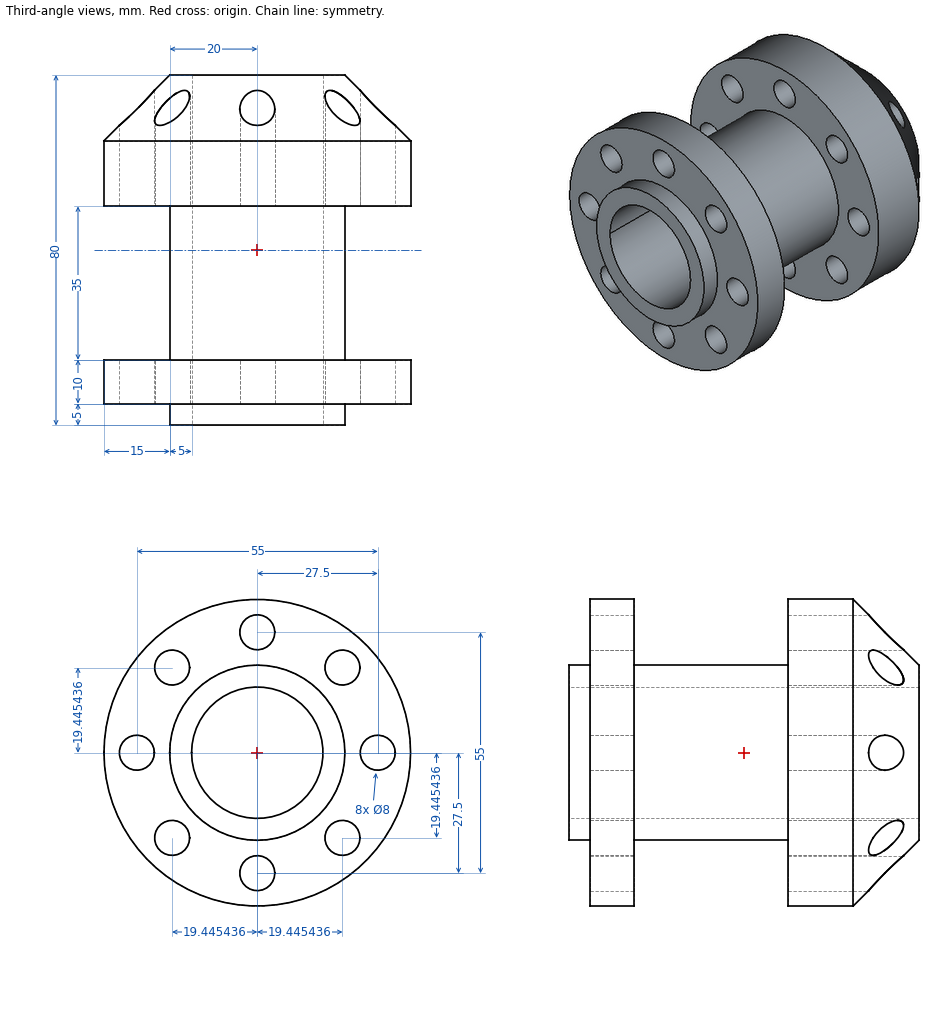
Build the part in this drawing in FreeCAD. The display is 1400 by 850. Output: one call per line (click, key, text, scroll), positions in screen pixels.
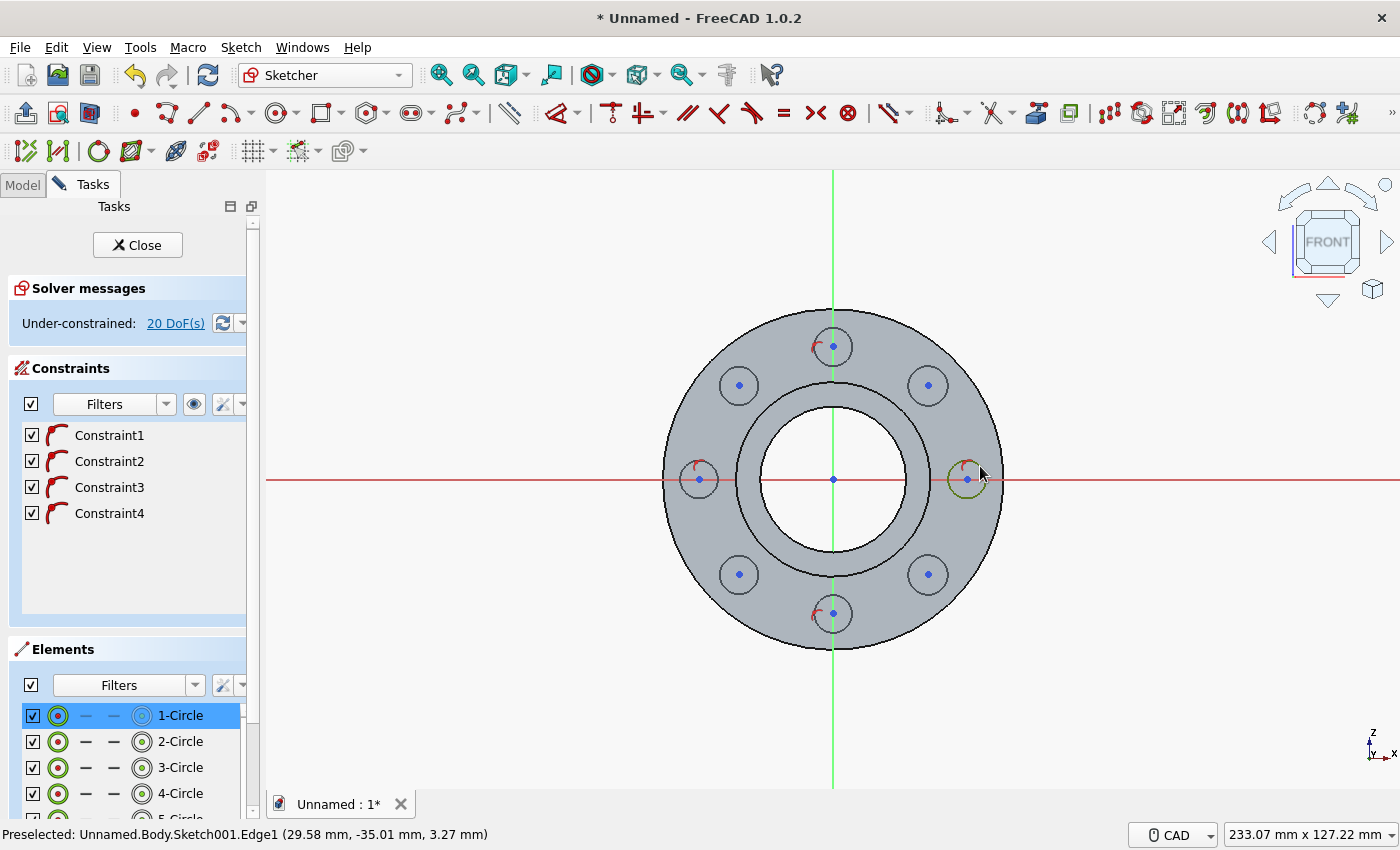
click(942, 561)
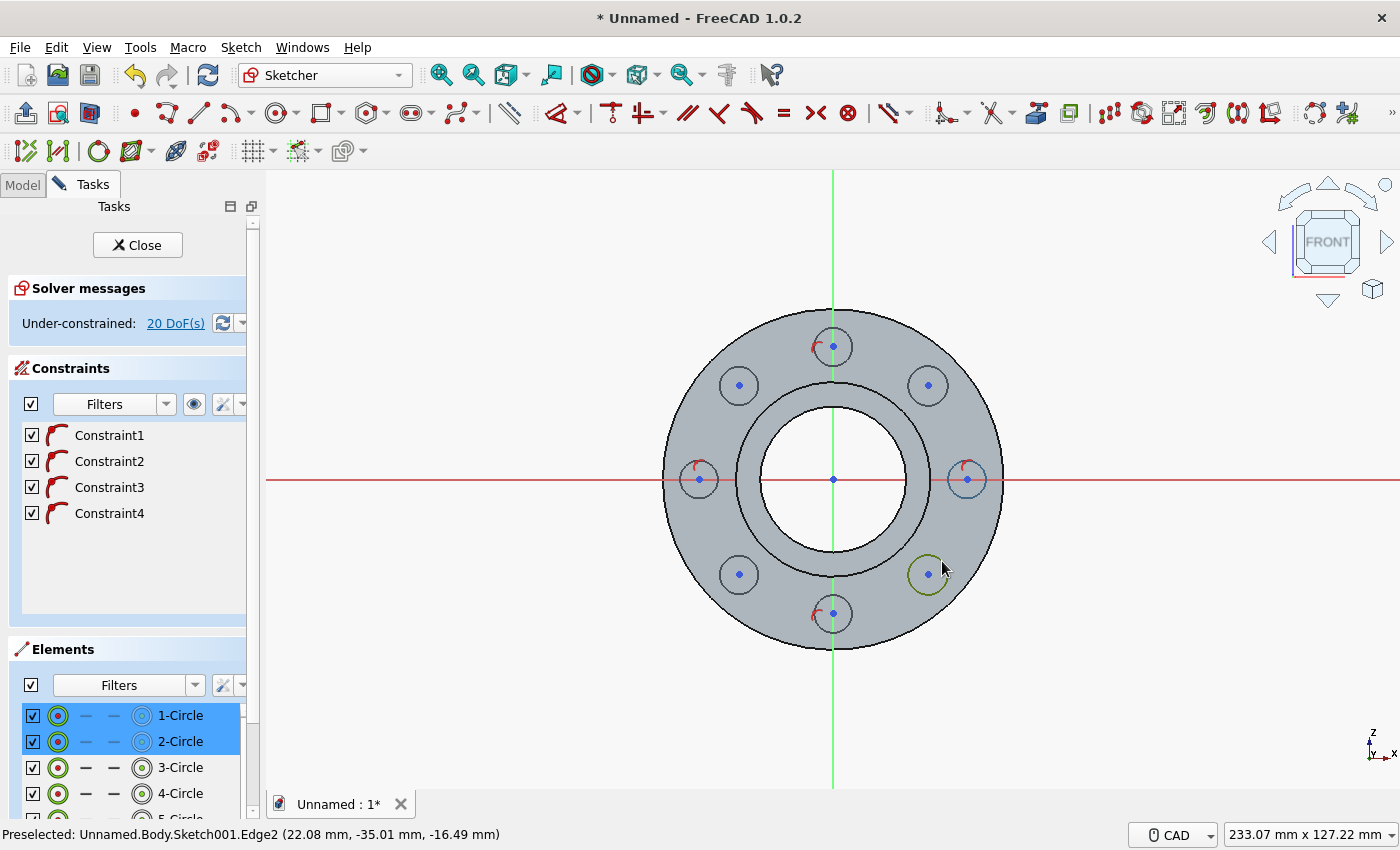
click(846, 601)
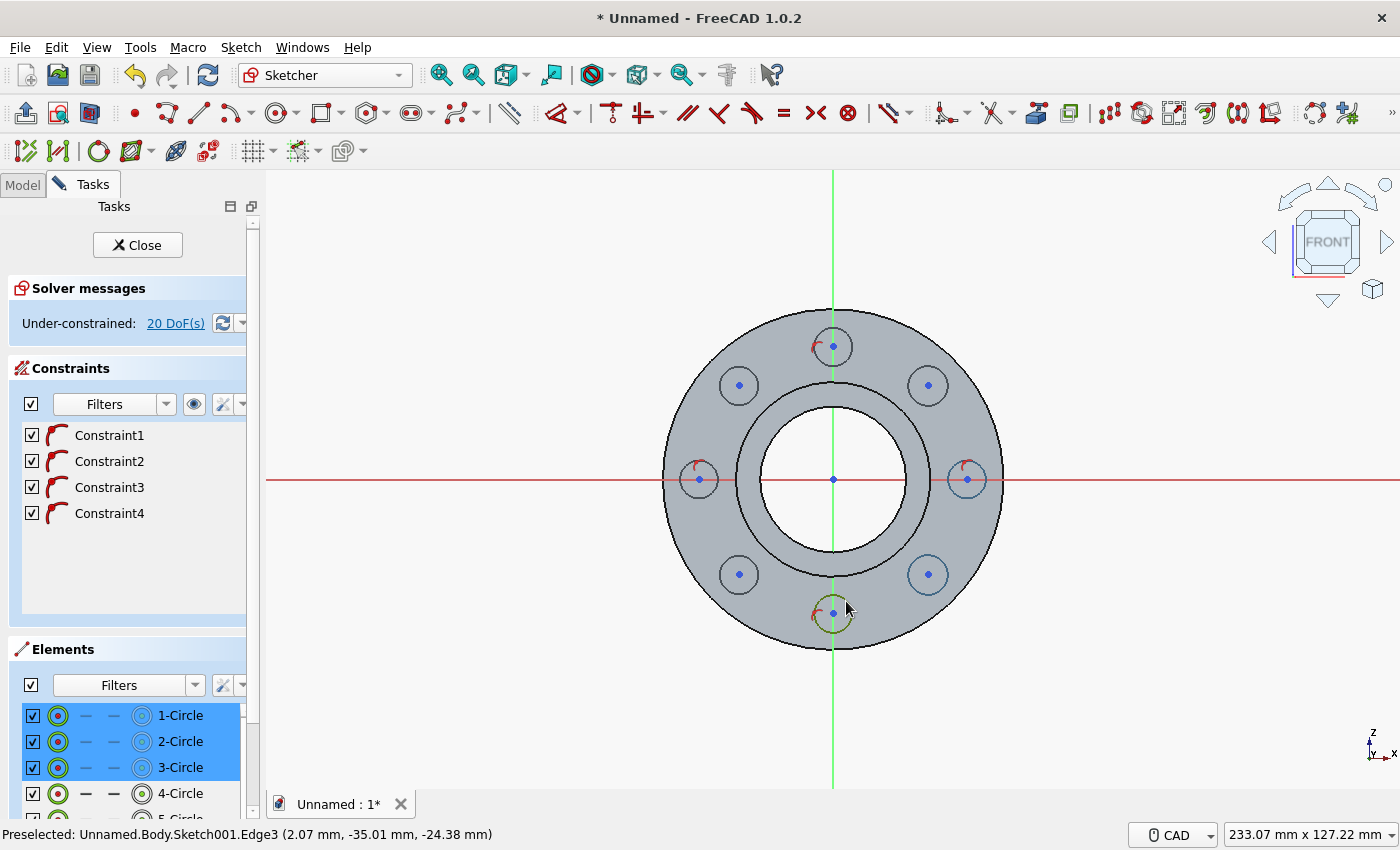
click(752, 561)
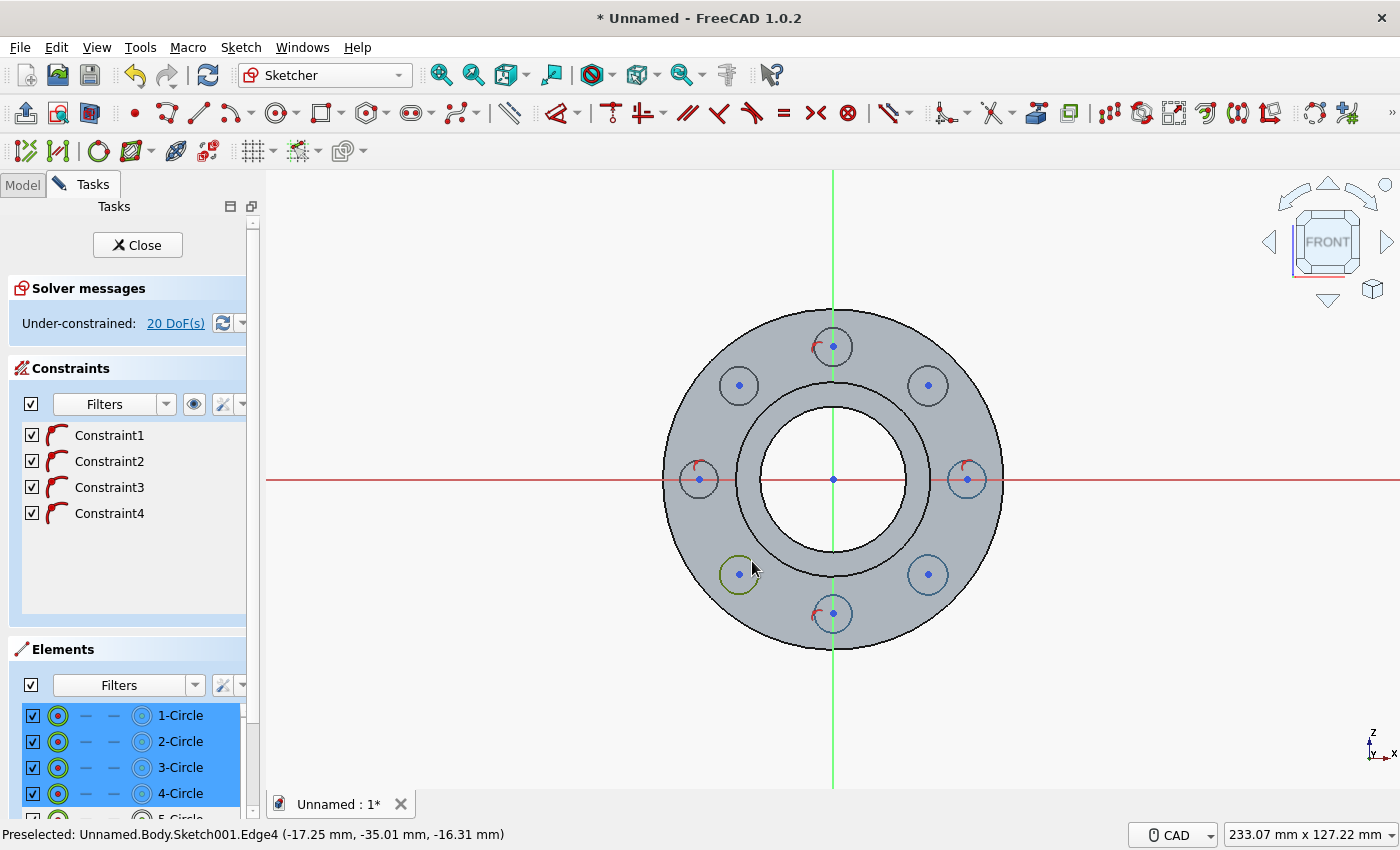
click(712, 466)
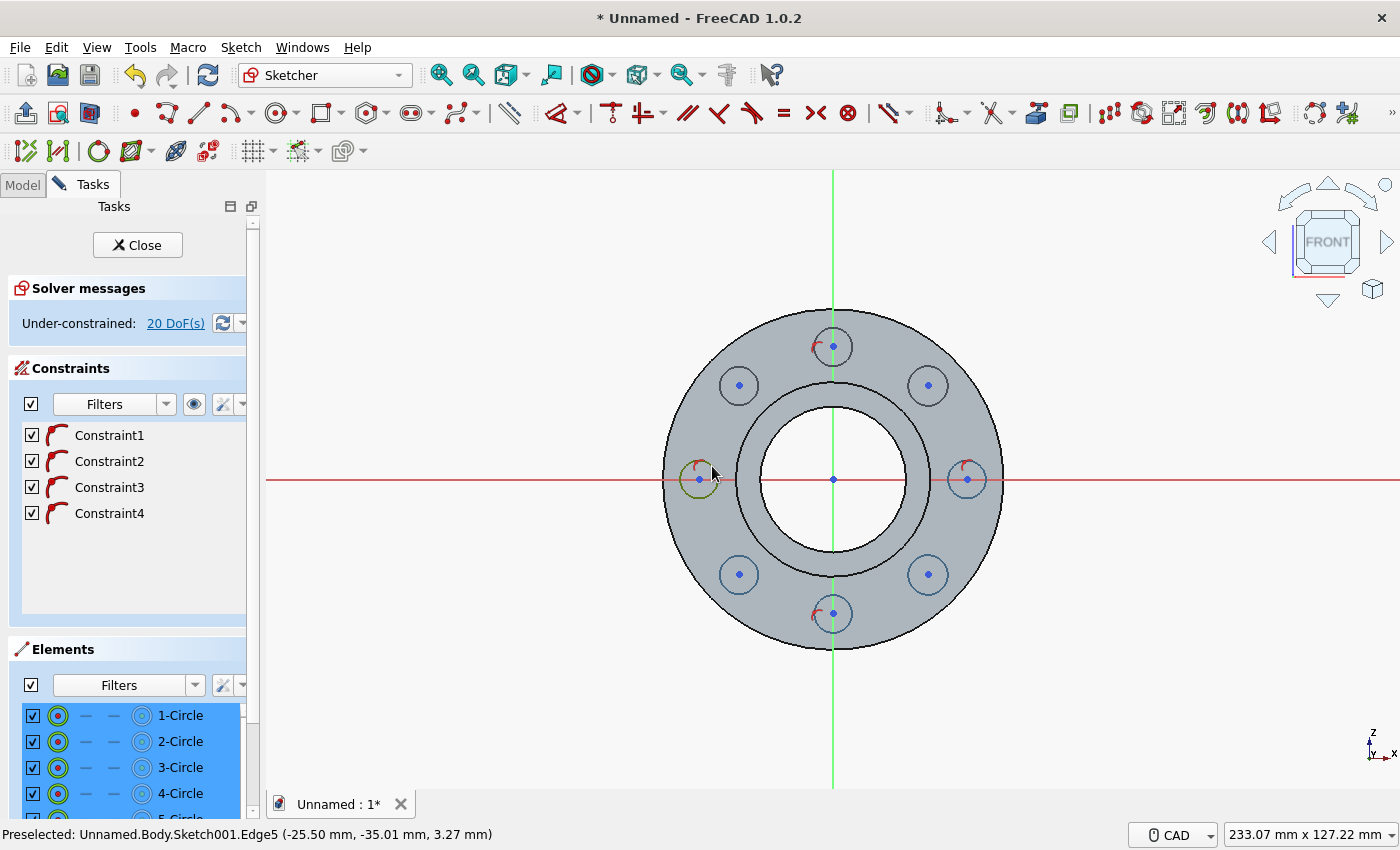
click(752, 372)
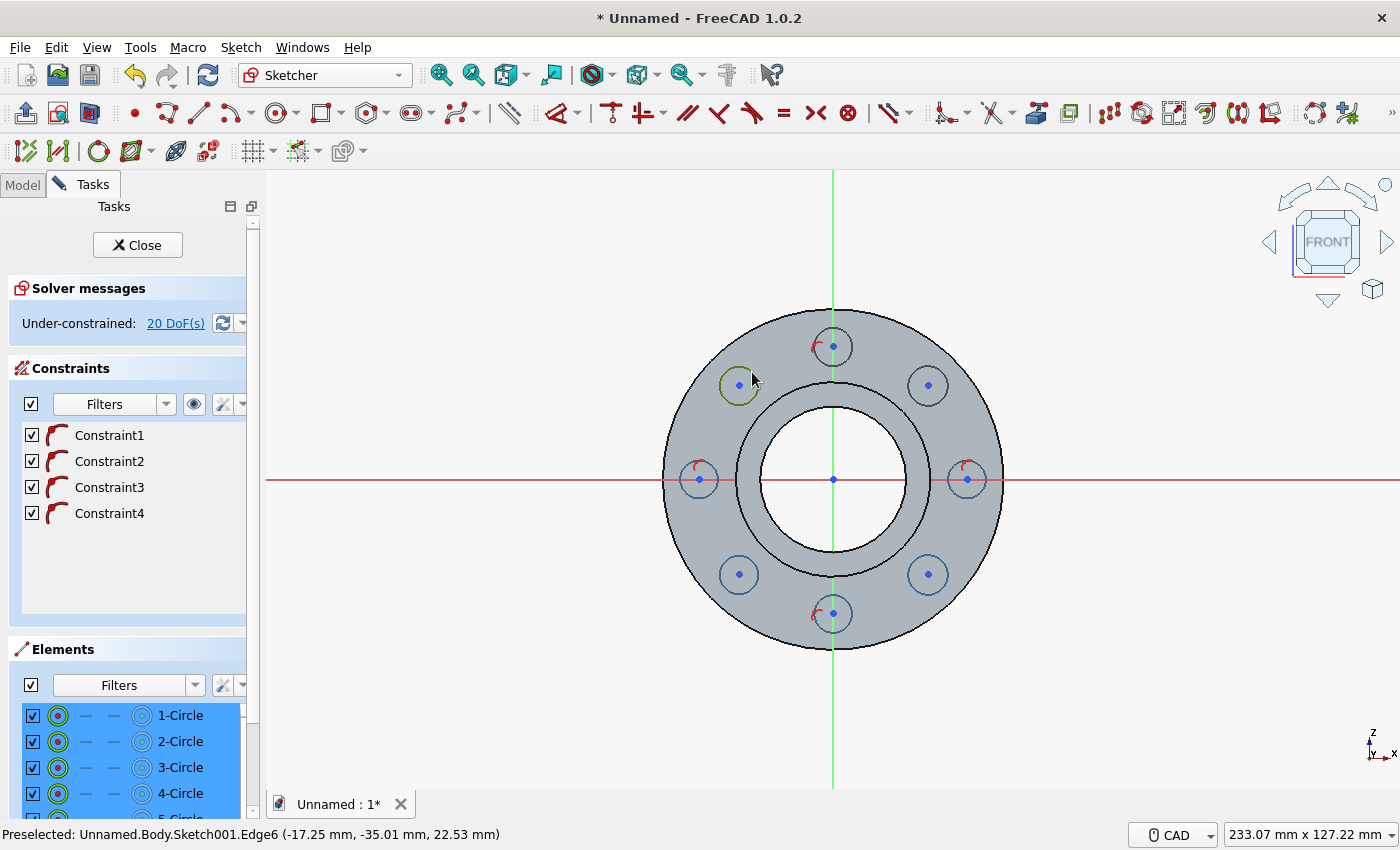
click(847, 333)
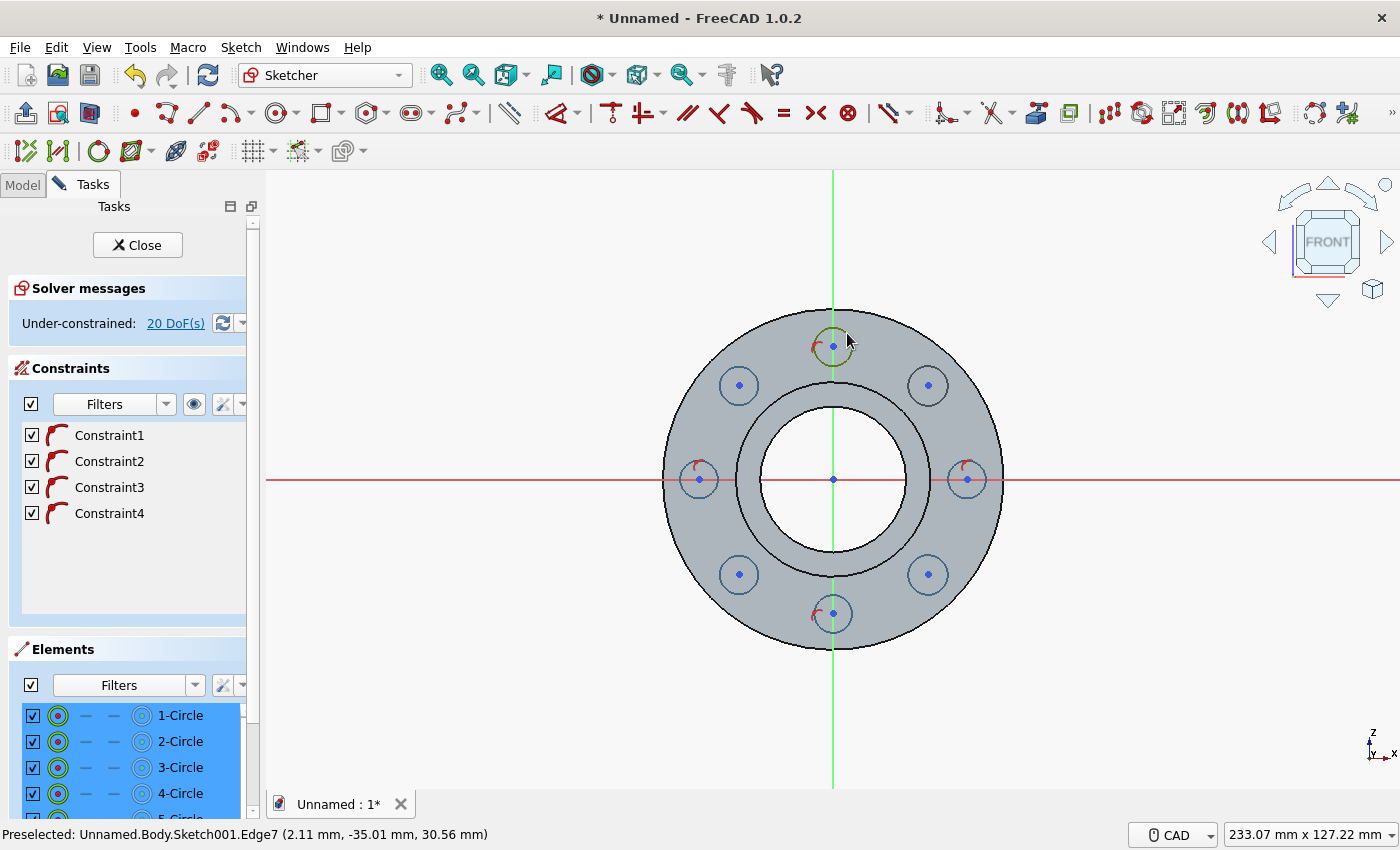
click(942, 372)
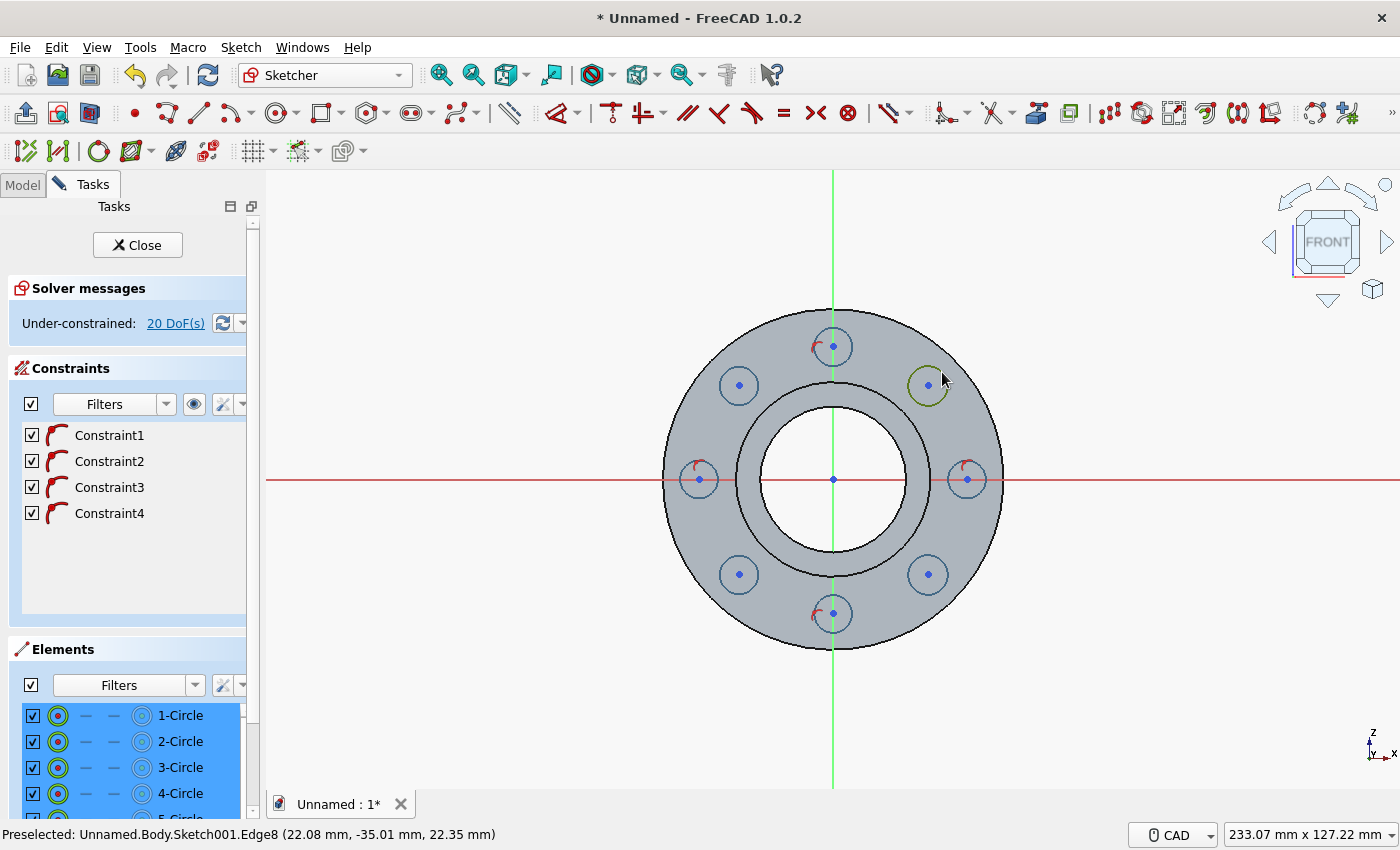
key(e)